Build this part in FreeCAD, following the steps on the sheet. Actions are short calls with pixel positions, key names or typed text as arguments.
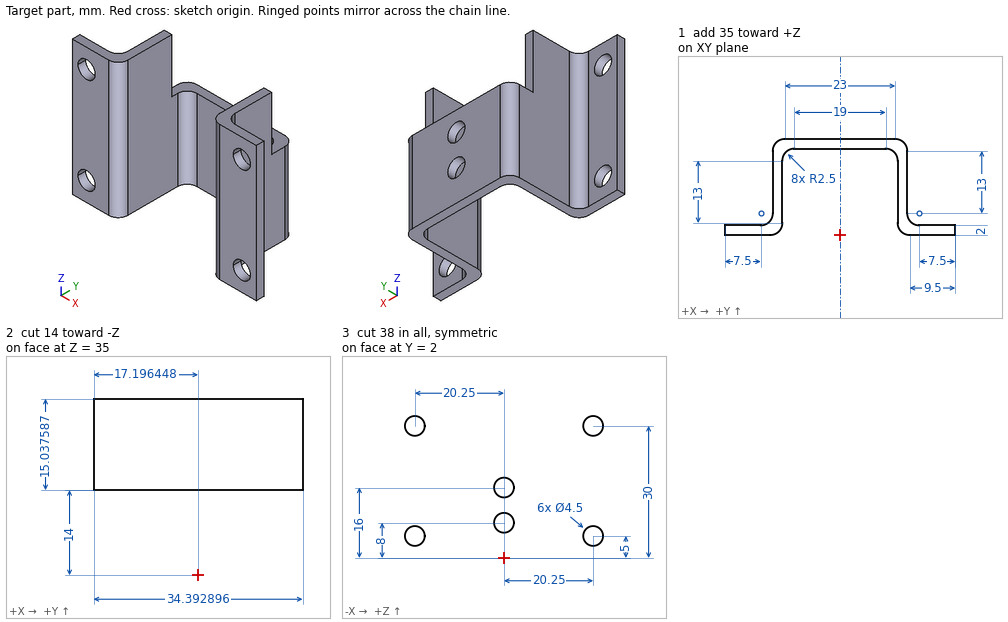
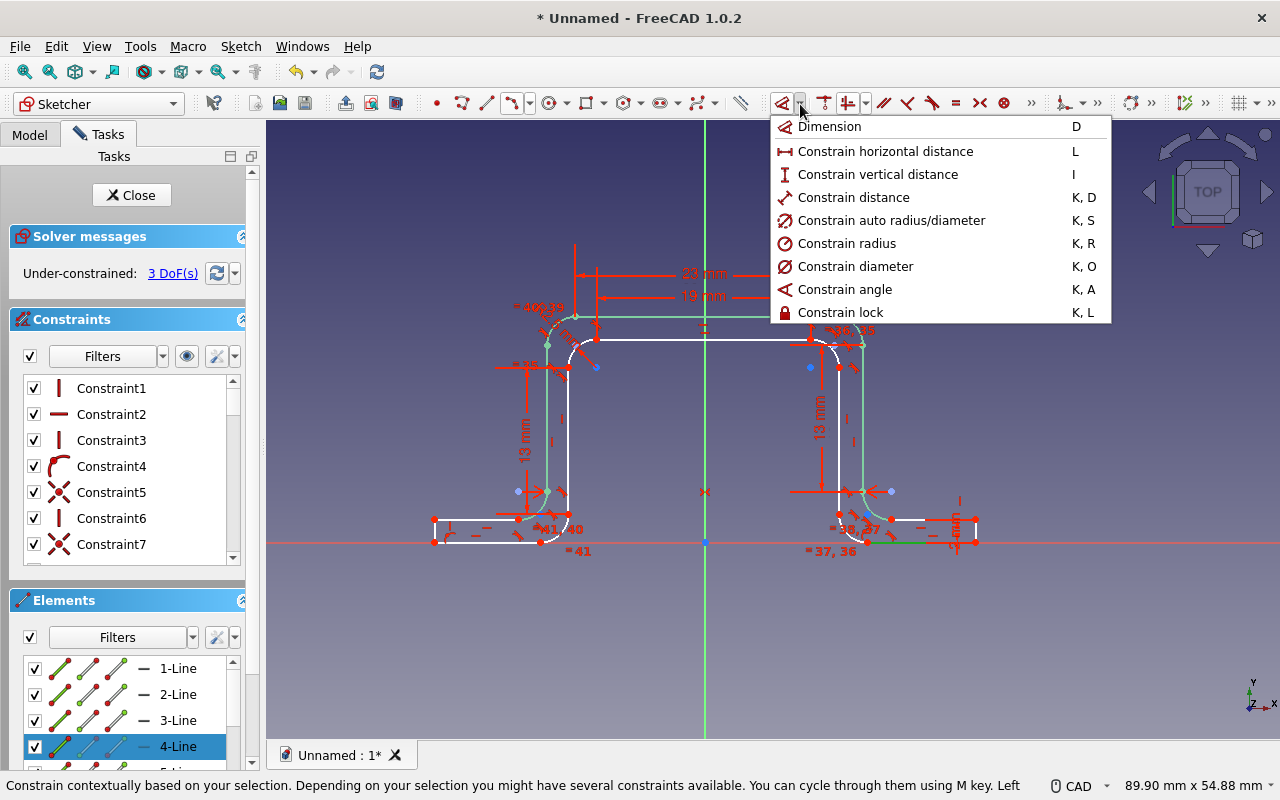
click(941, 152)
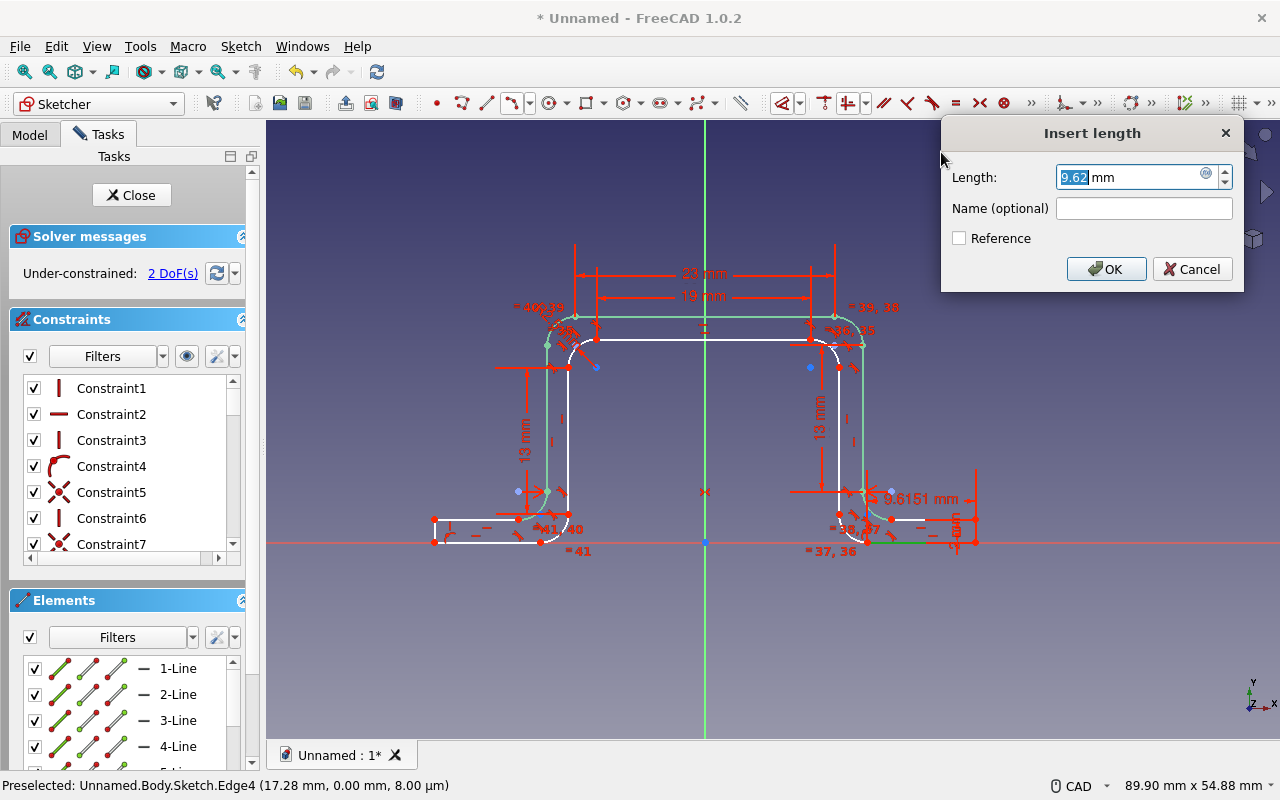
text(9.5)
key(Return)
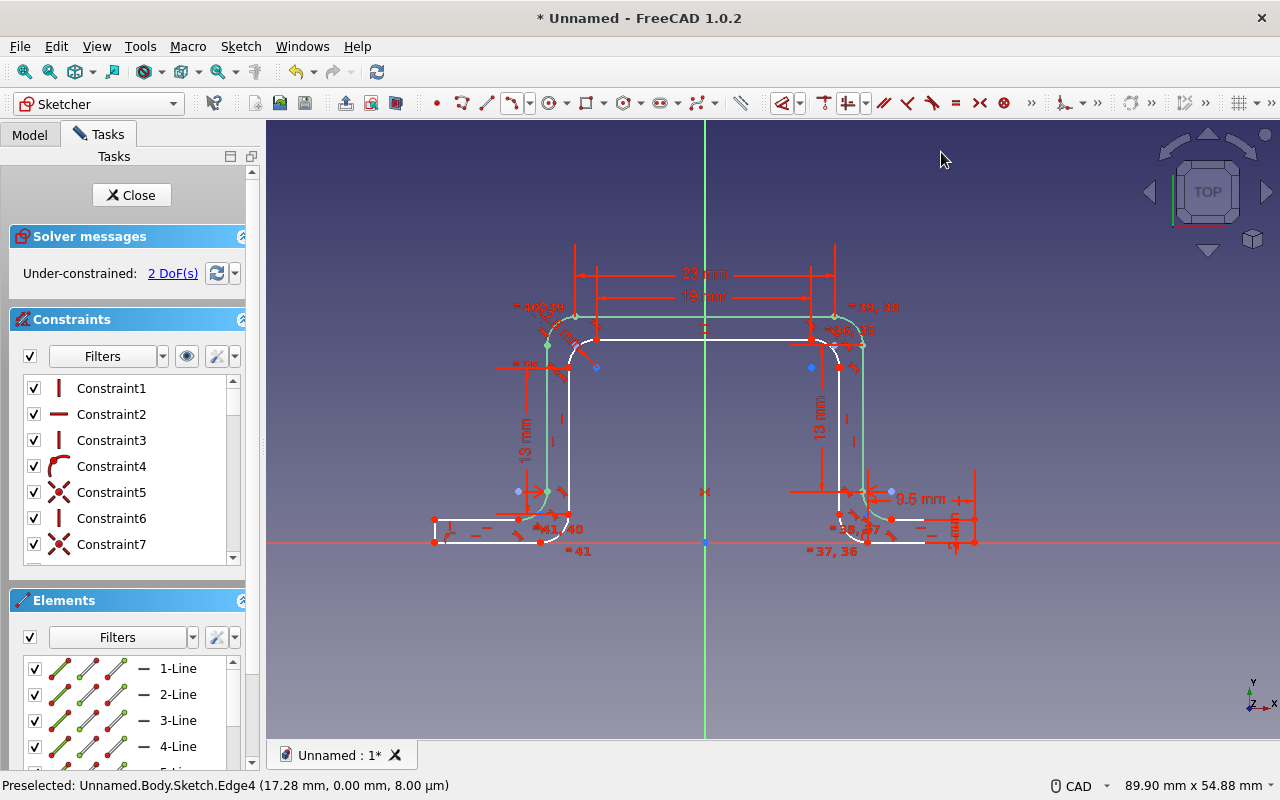
click(916, 520)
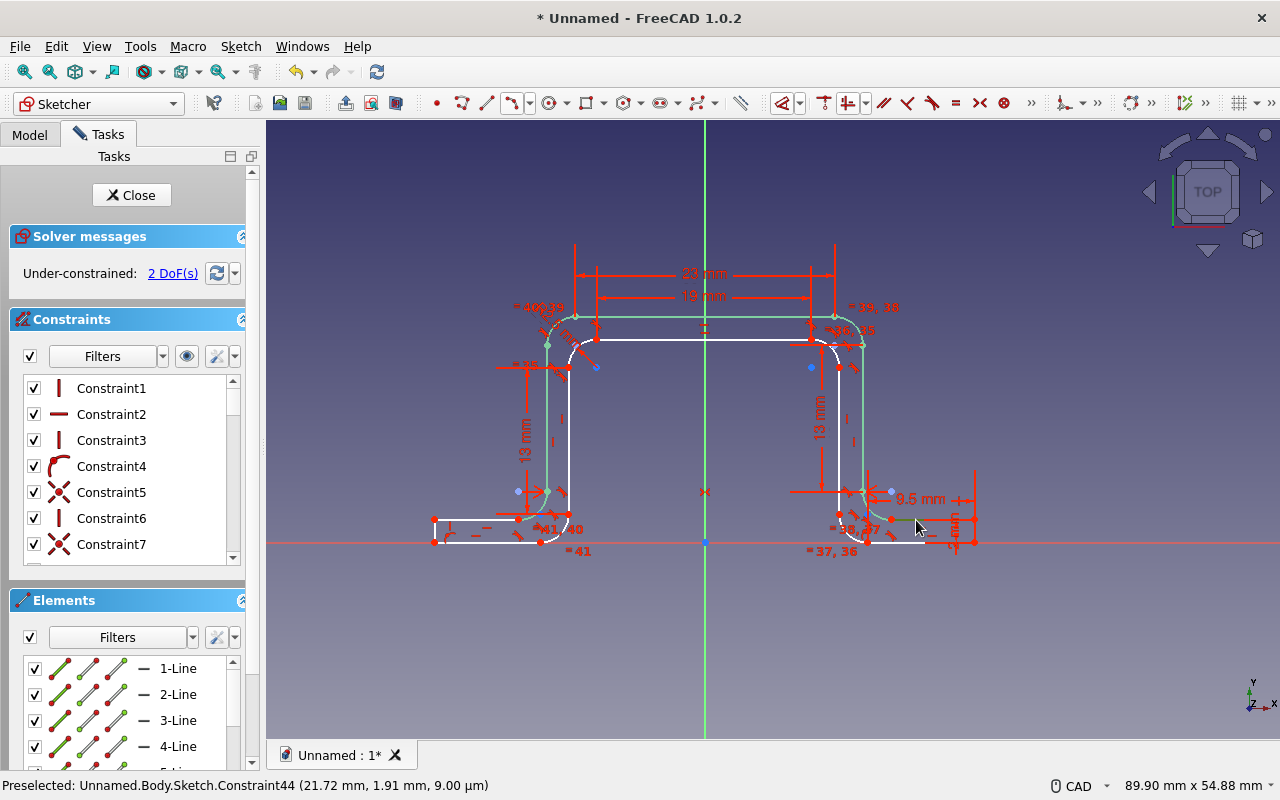
key(l)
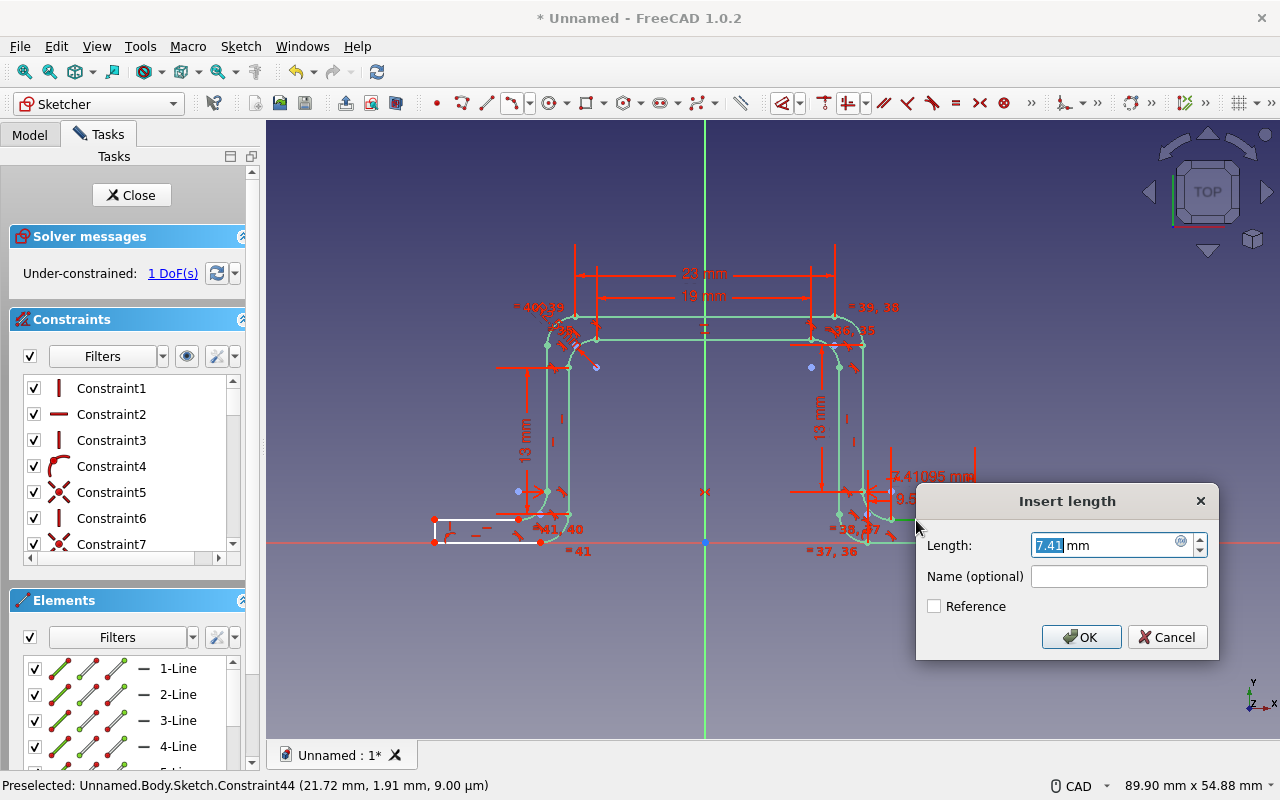
text(7.5)
key(Return)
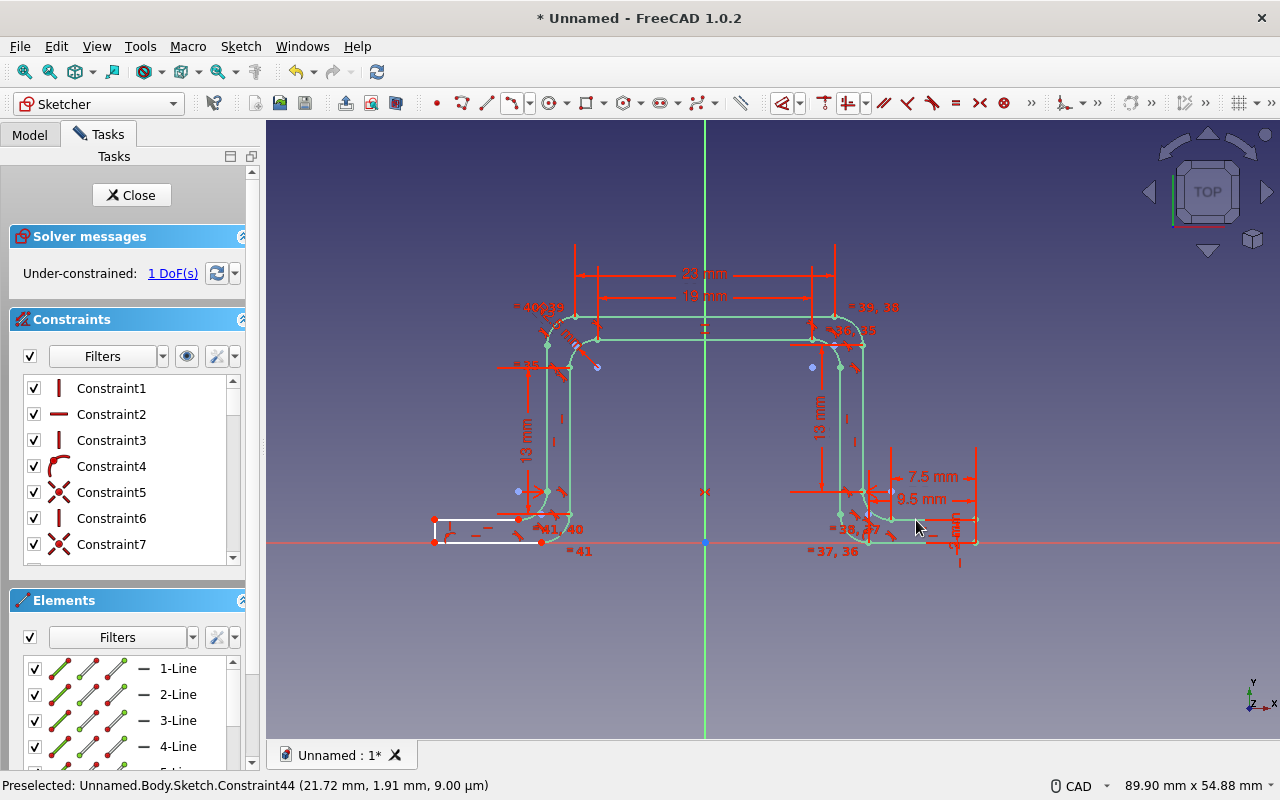
click(494, 520)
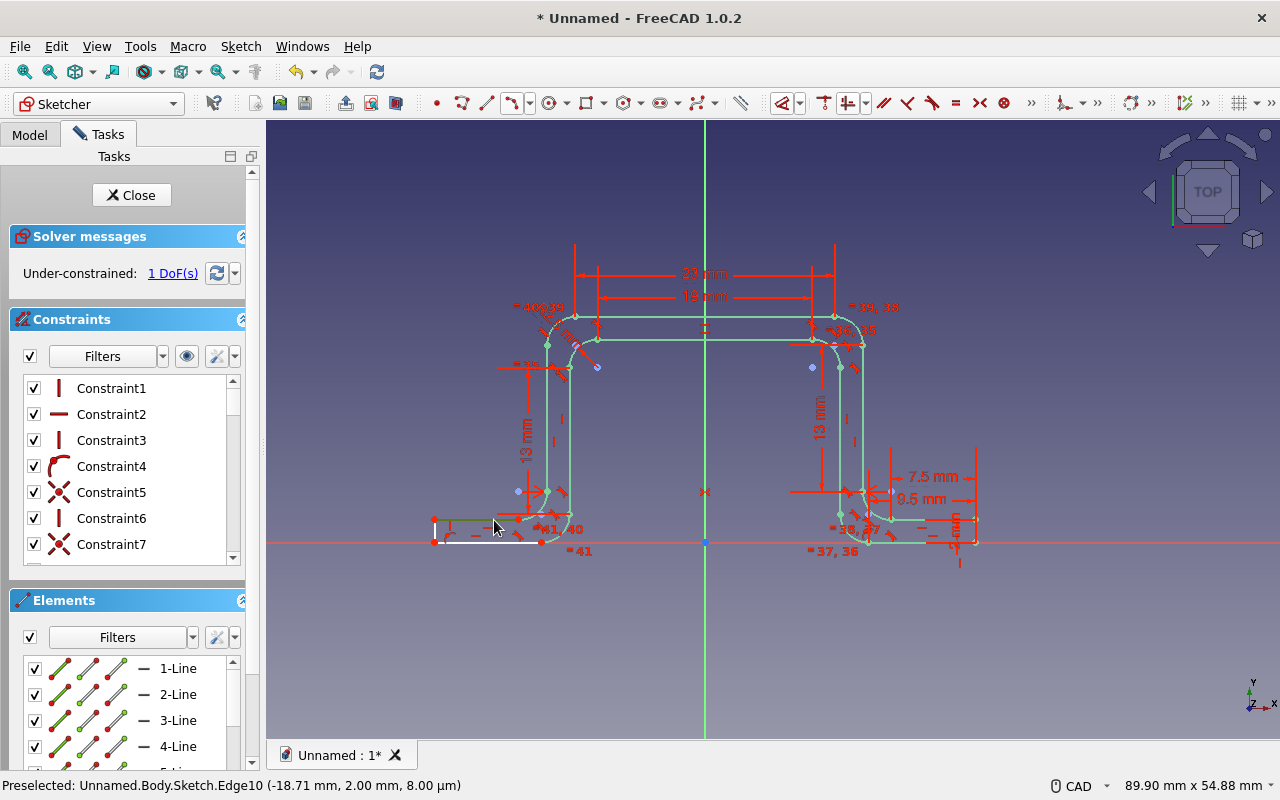
key(l)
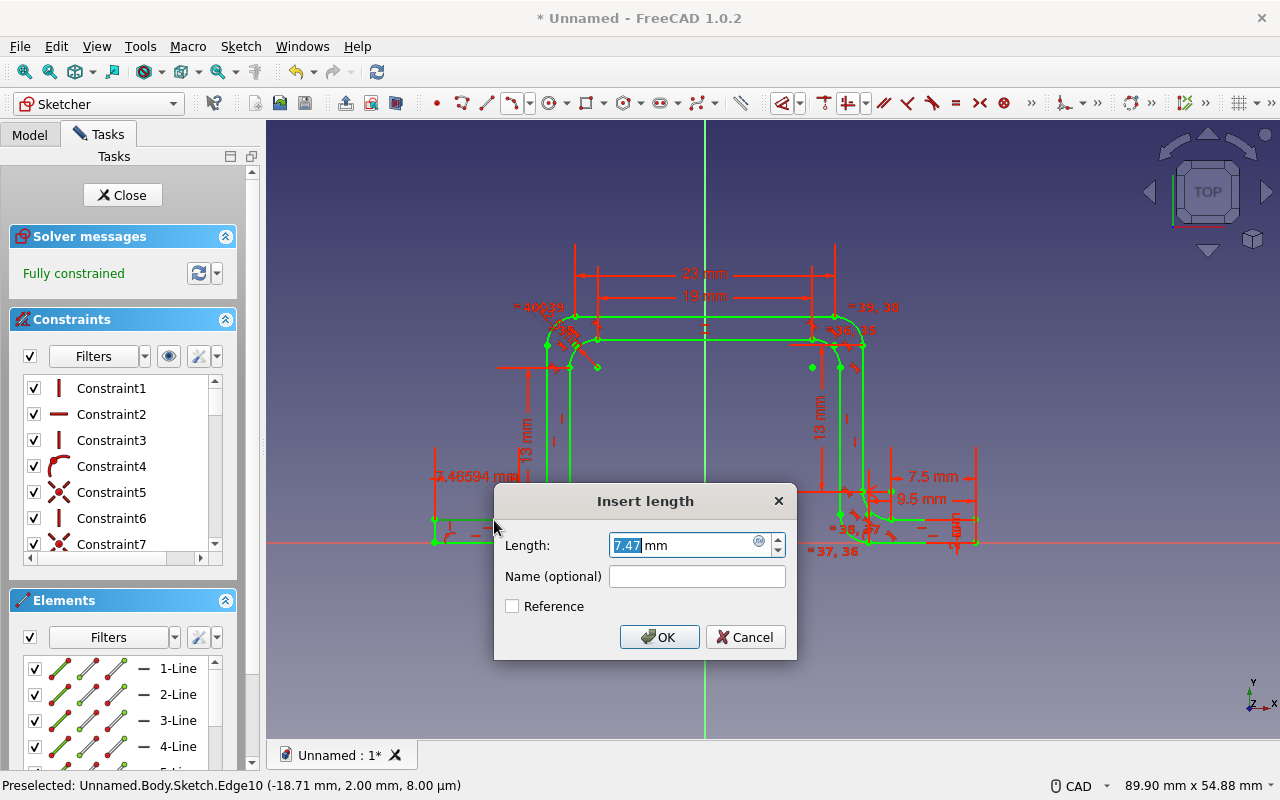
text(7.5)
key(Return)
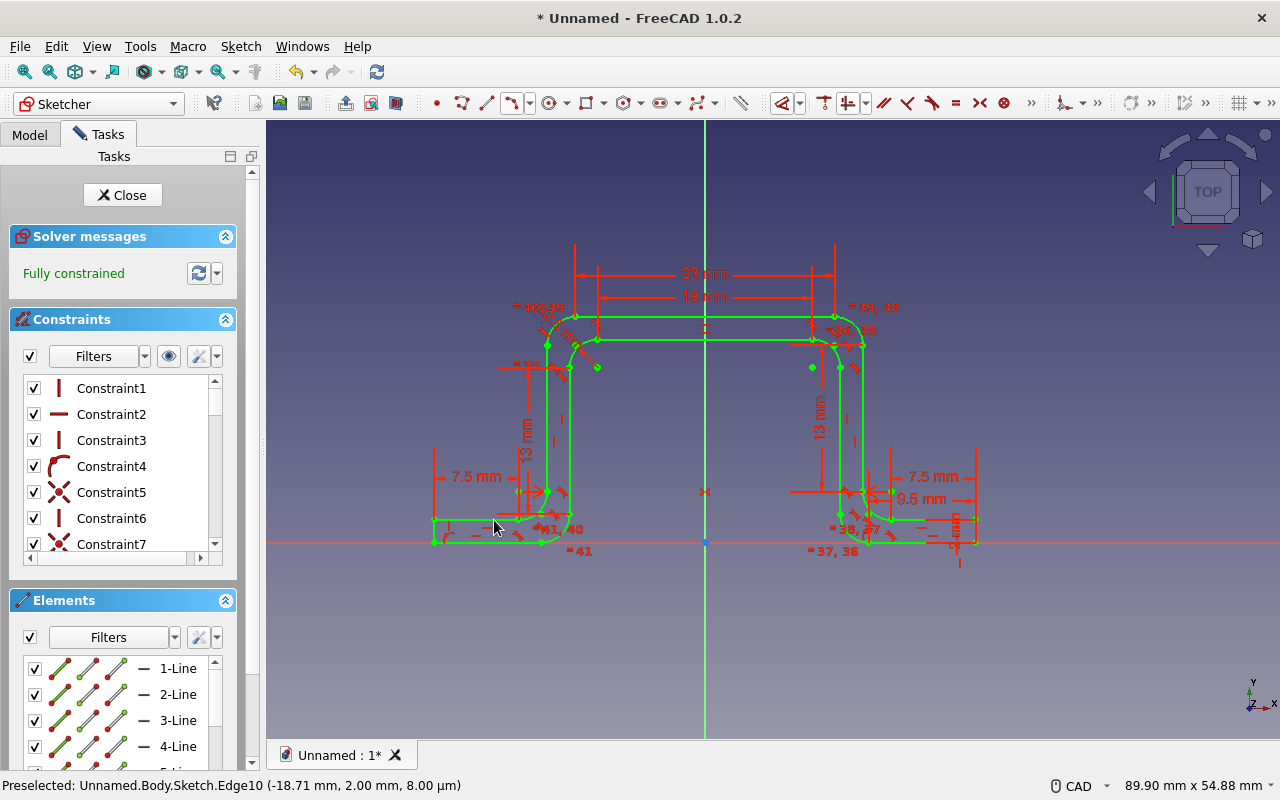
click(123, 195)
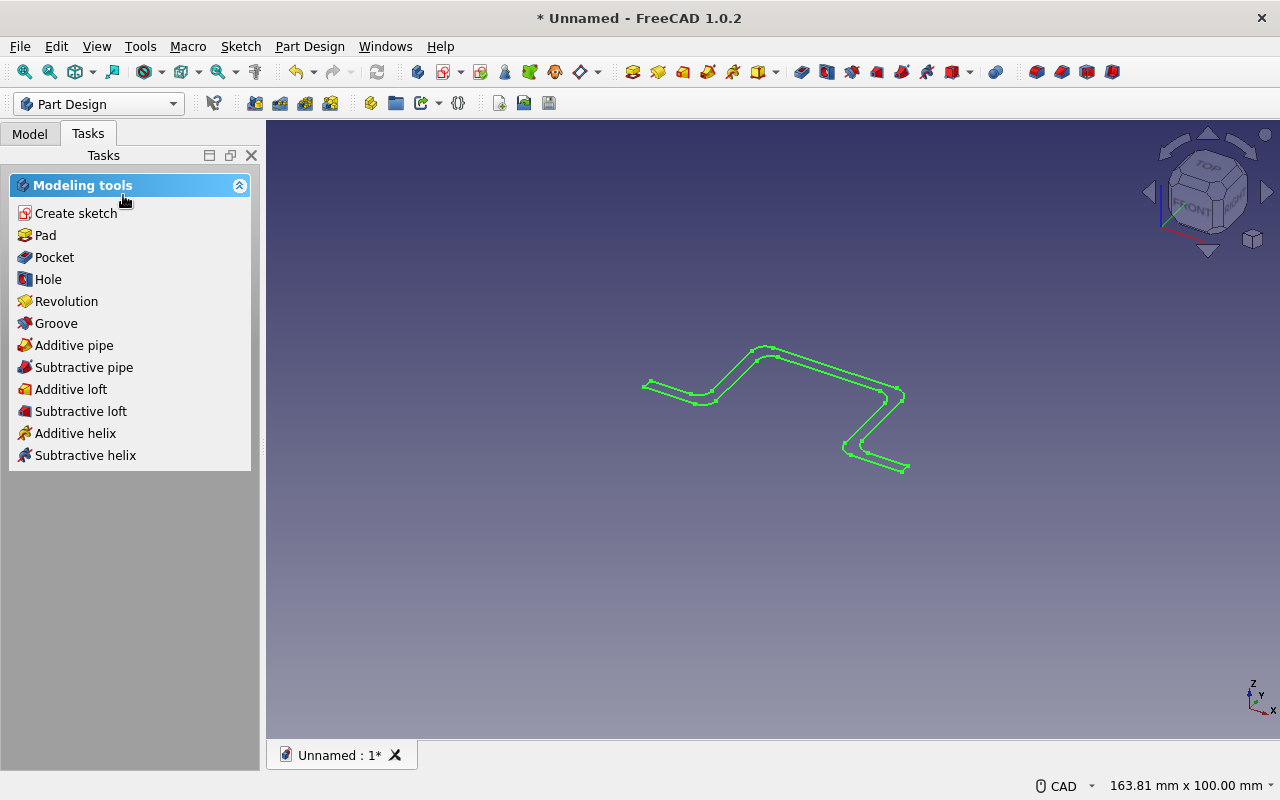
click(633, 72)